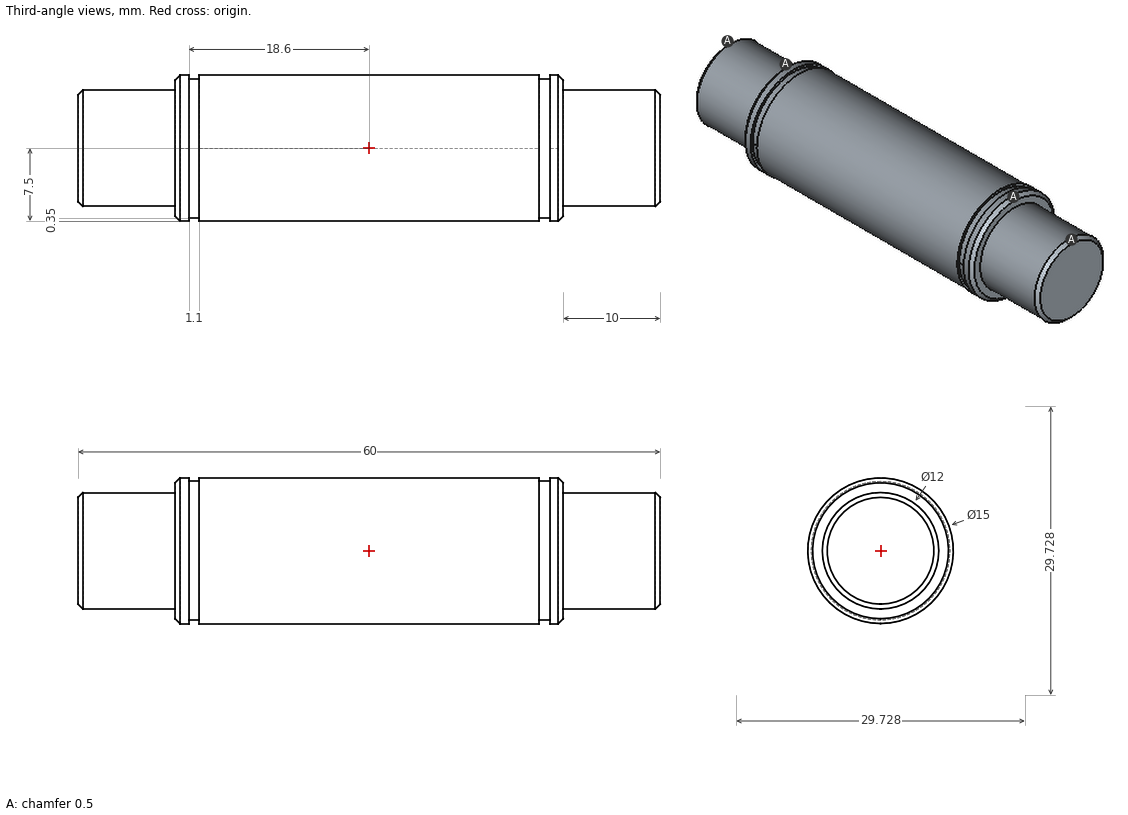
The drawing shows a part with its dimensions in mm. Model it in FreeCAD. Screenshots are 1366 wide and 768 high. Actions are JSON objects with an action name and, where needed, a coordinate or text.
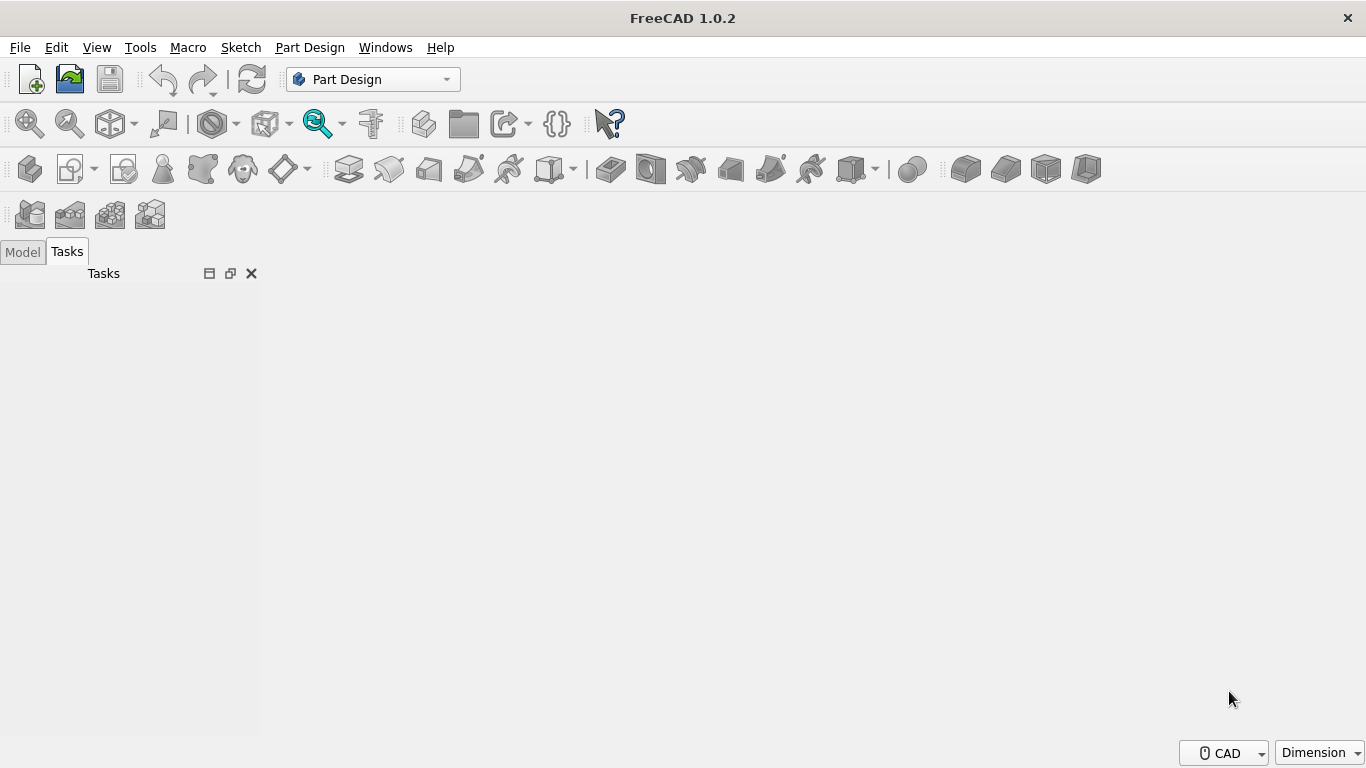
{"action": "key", "text": "ctrl+n"}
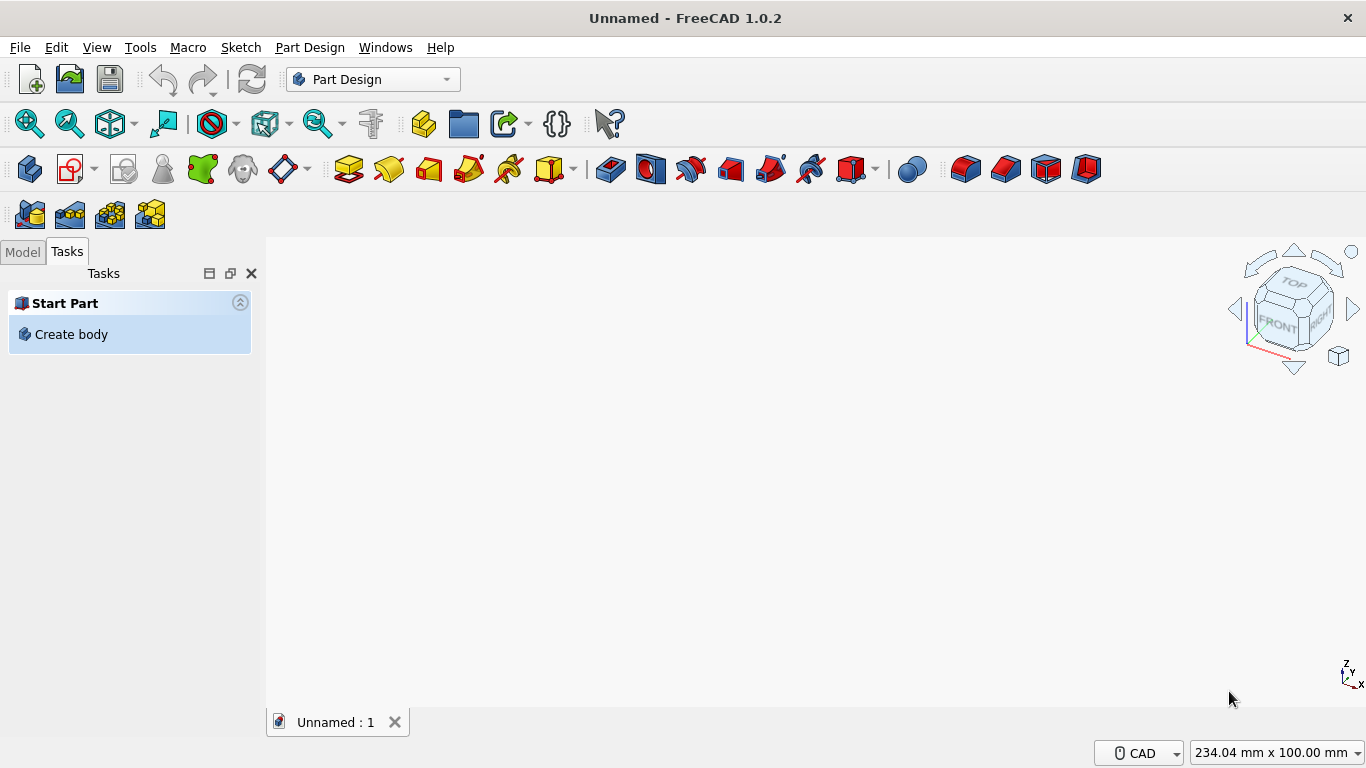
{"action": "left_click", "coordinate": [70, 170]}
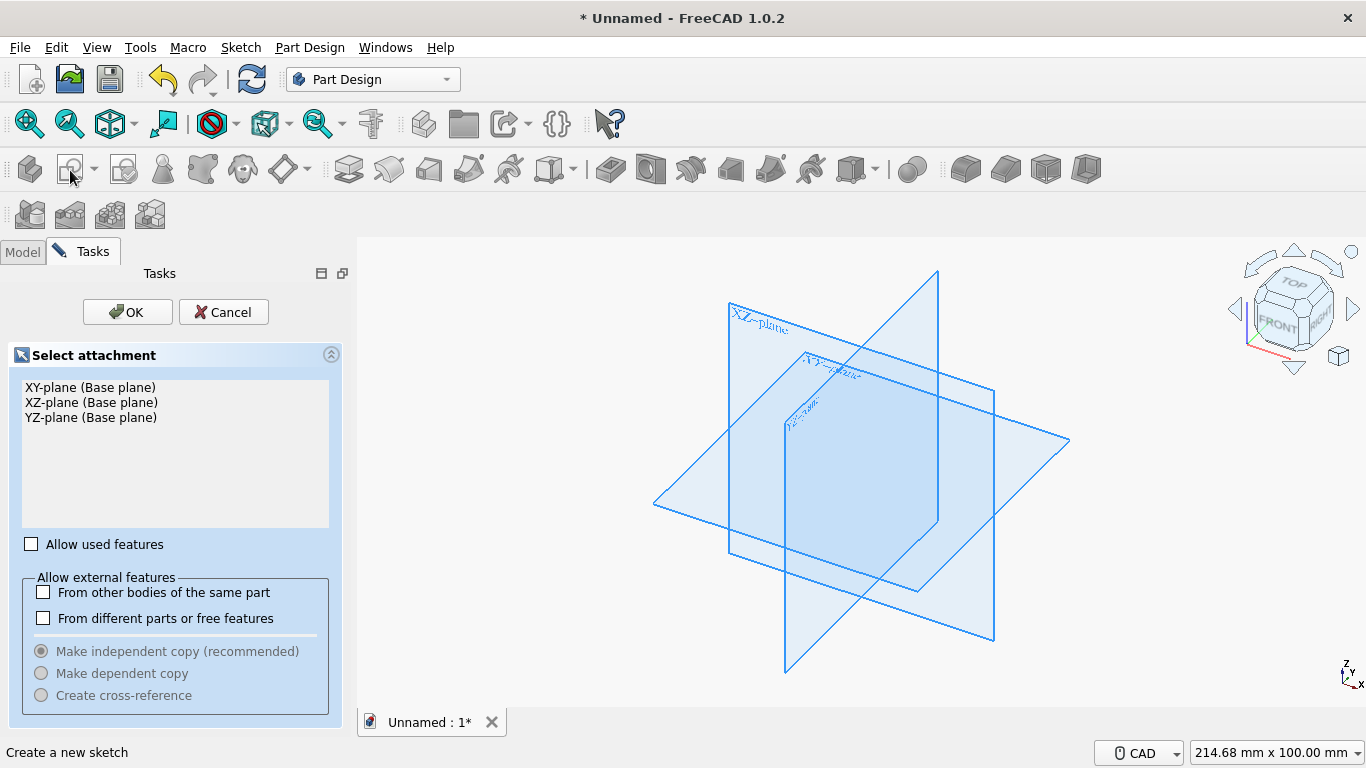
{"action": "left_click", "coordinate": [82, 418]}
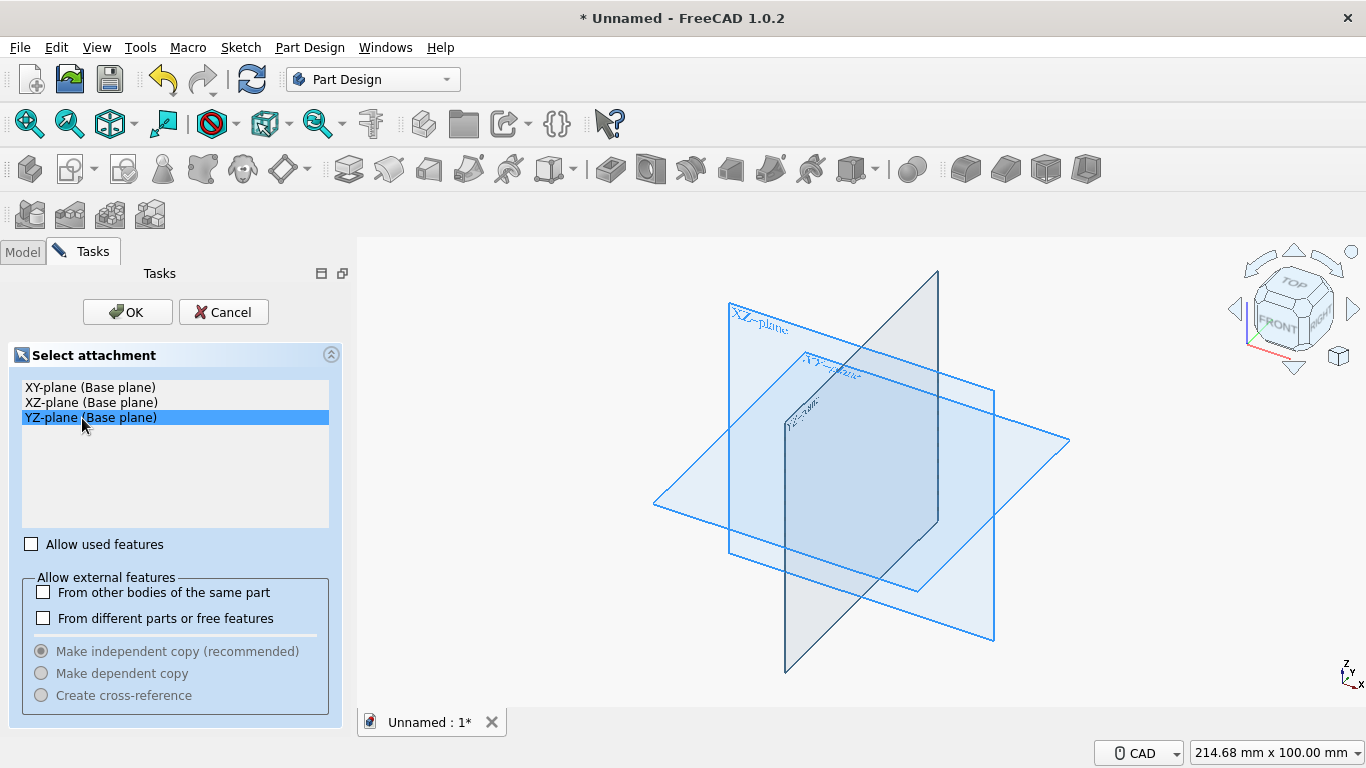
{"action": "left_click", "coordinate": [128, 312]}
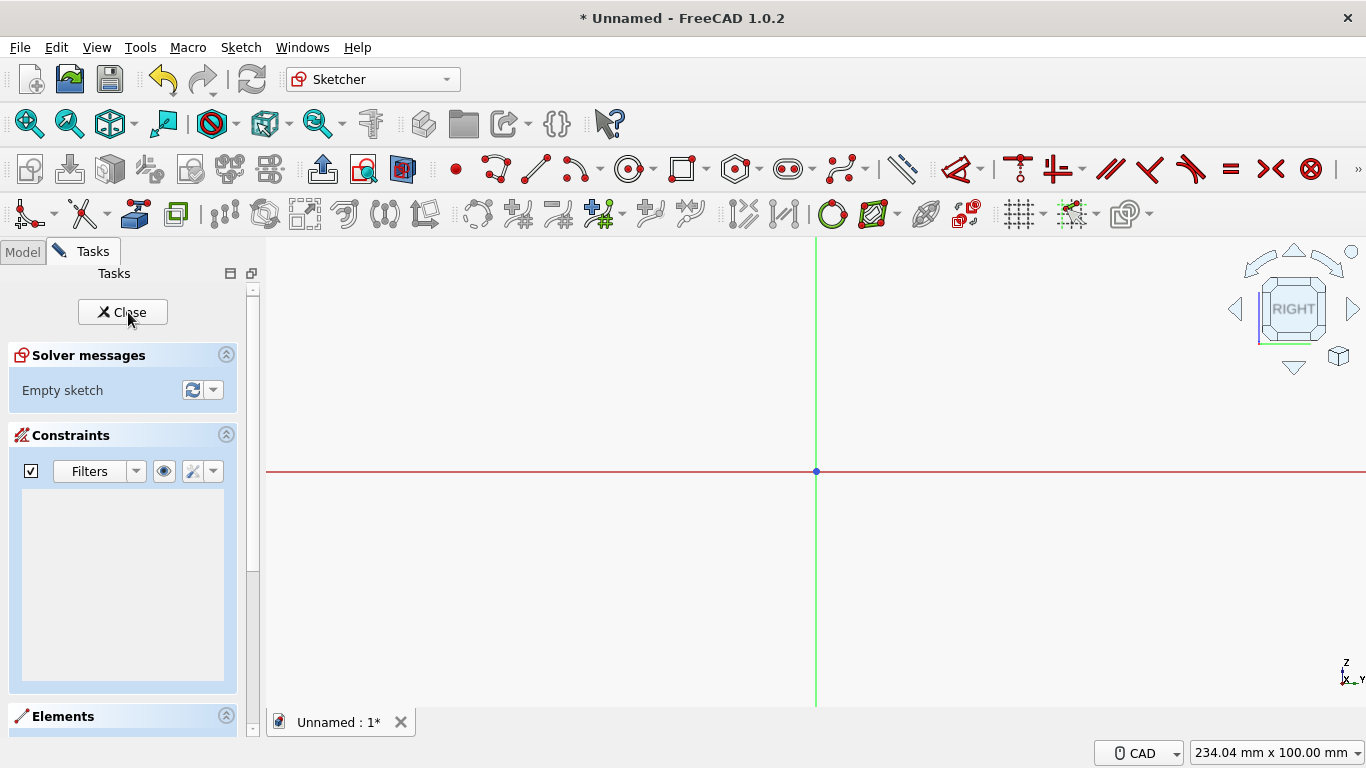
{"action": "scroll", "coordinate": [838, 472], "scroll_direction": "up", "scroll_amount": 7}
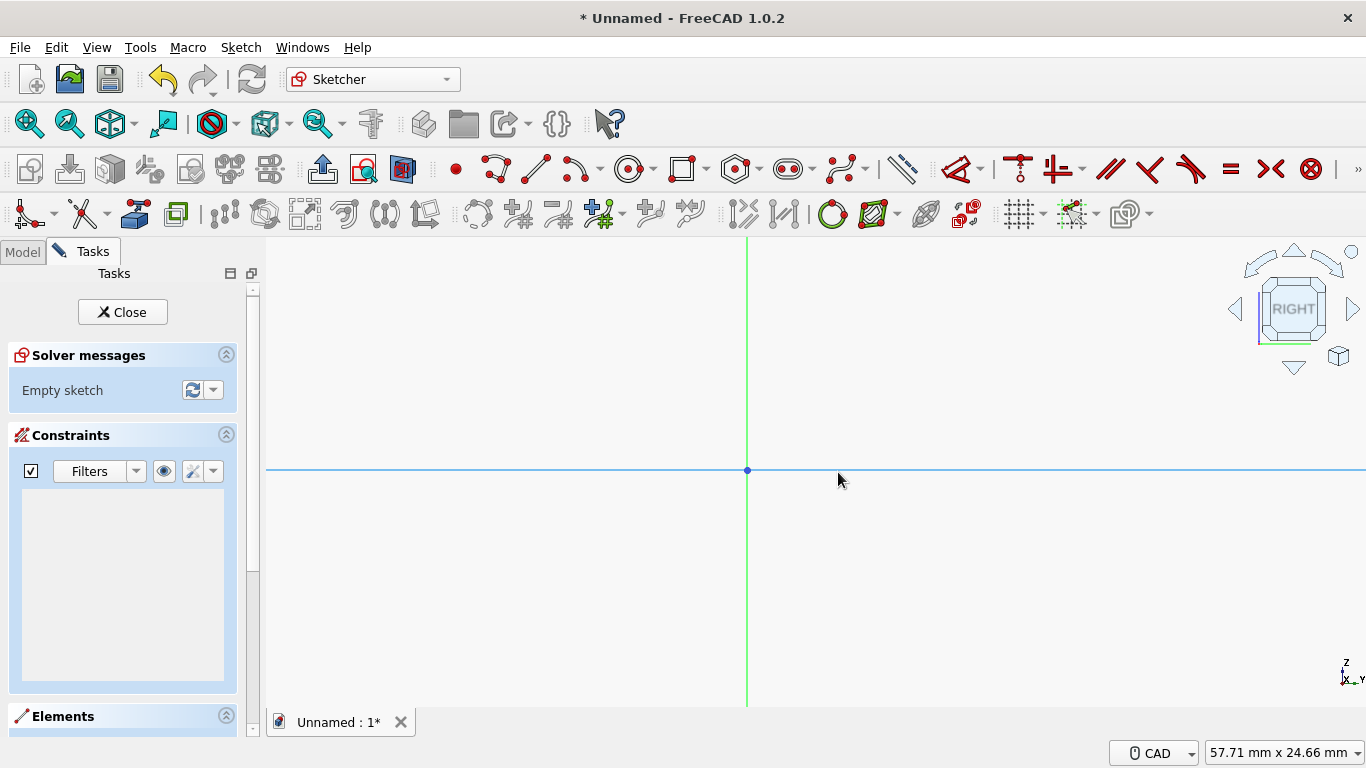
{"action": "key", "text": "g c"}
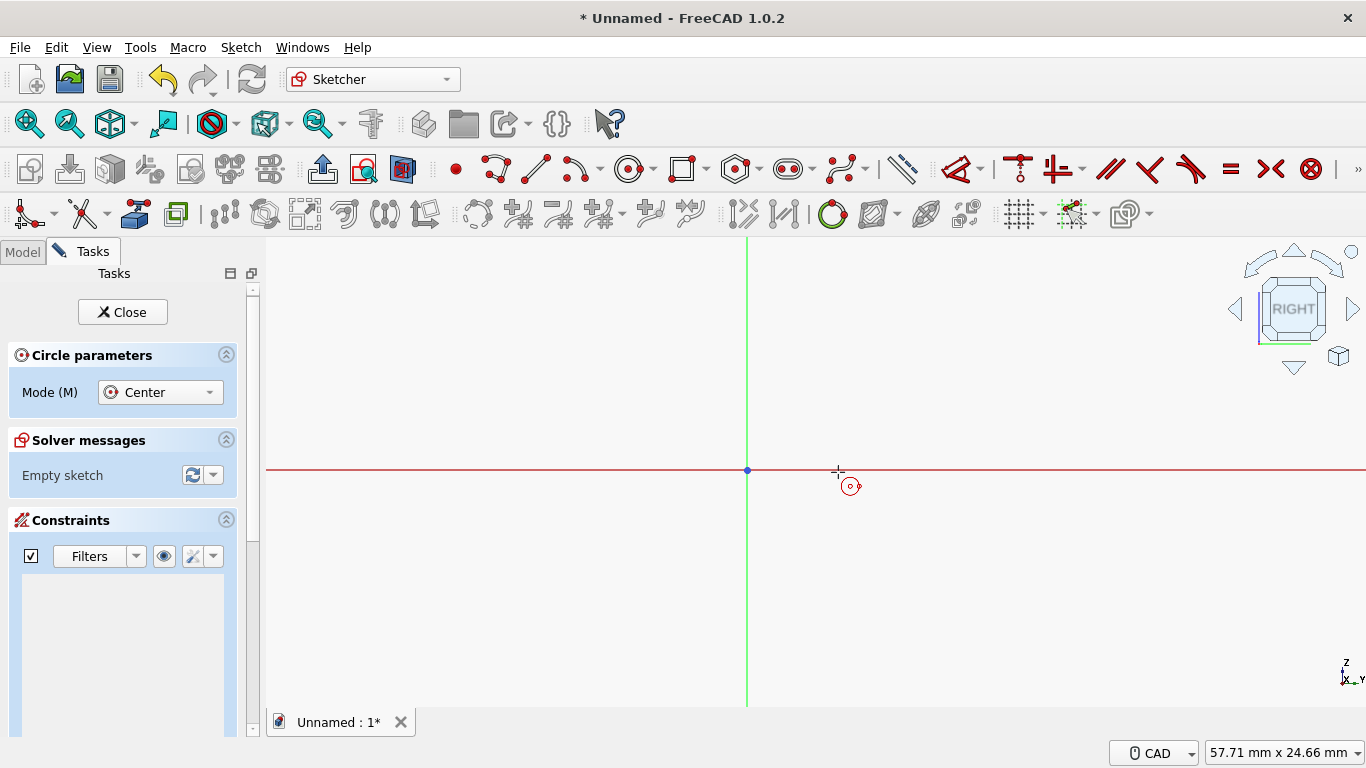
{"action": "left_click", "coordinate": [747, 470]}
{"action": "left_click", "coordinate": [848, 369]}
{"action": "key", "text": "Escape"}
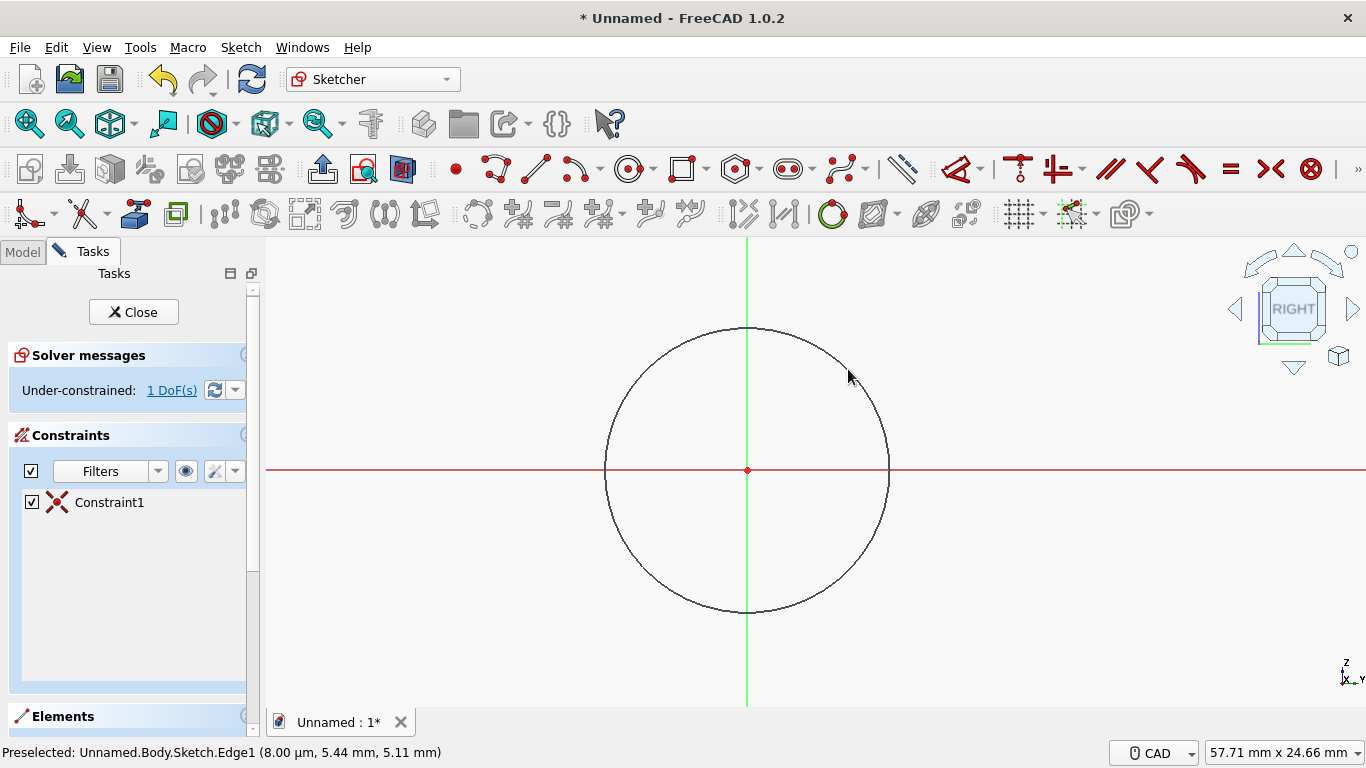
{"action": "left_click", "coordinate": [956, 170]}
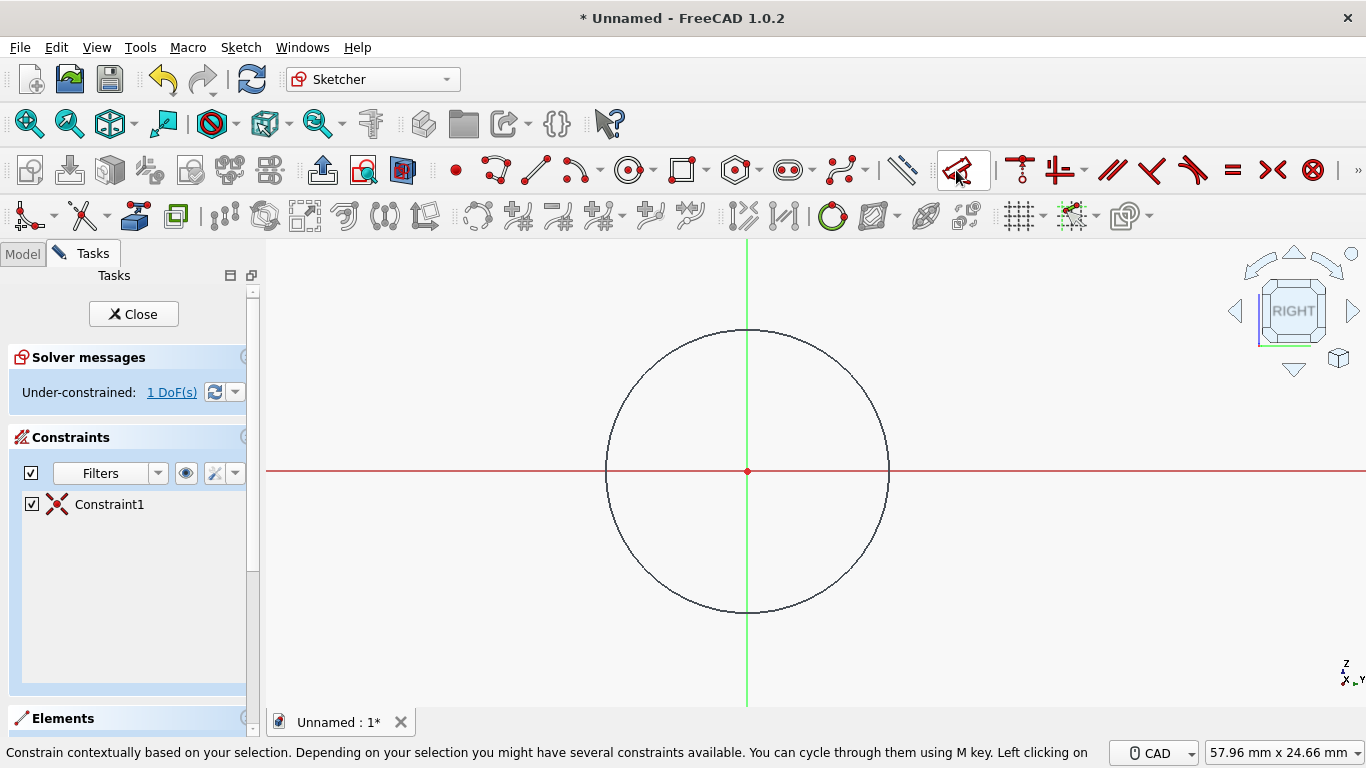
{"action": "left_click", "coordinate": [847, 371]}
{"action": "left_click", "coordinate": [870, 348]}